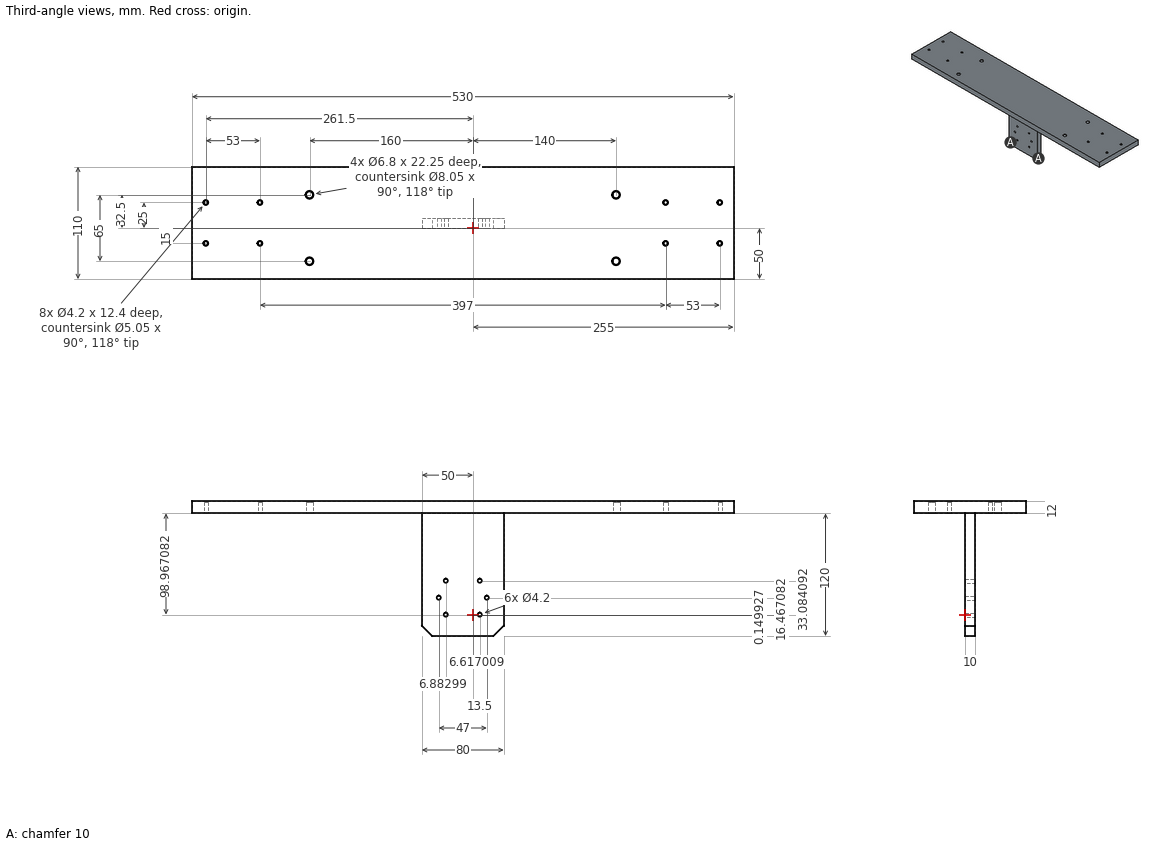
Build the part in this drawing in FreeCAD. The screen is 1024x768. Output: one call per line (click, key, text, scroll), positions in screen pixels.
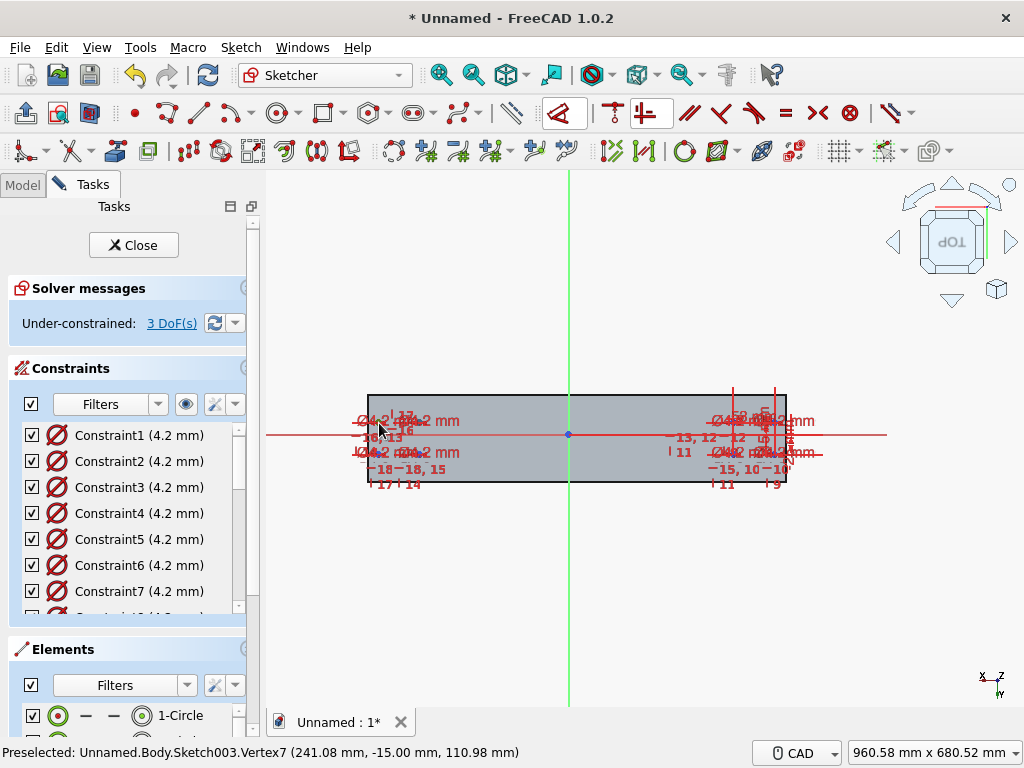
key(l)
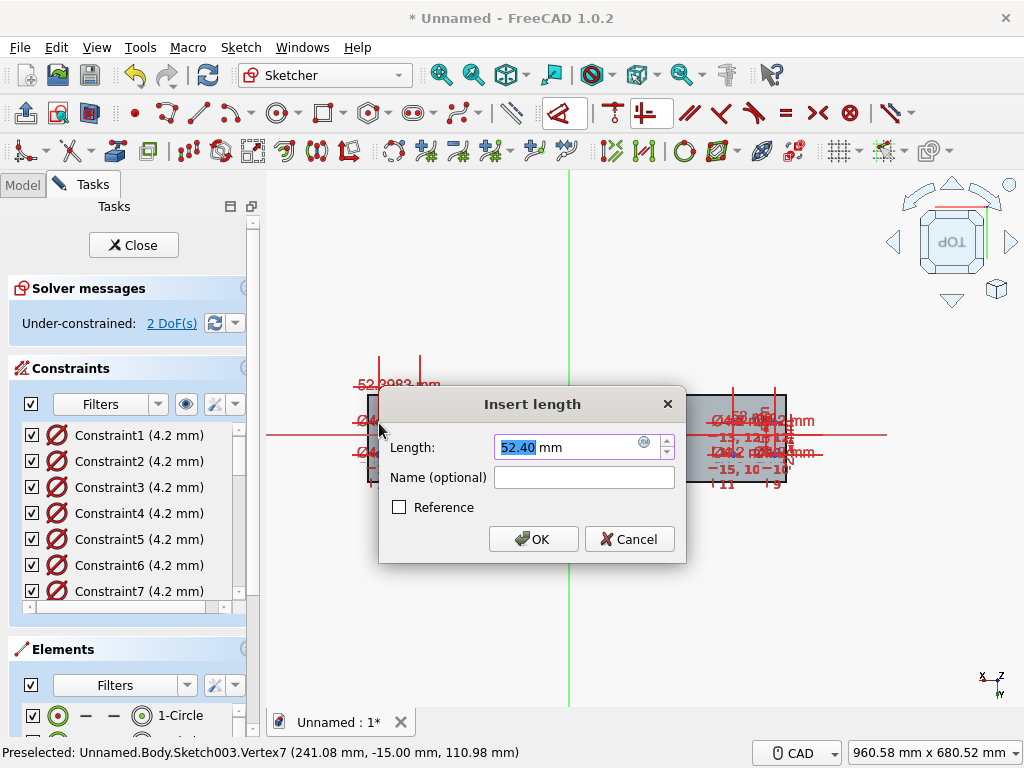
text(53)
key(Return)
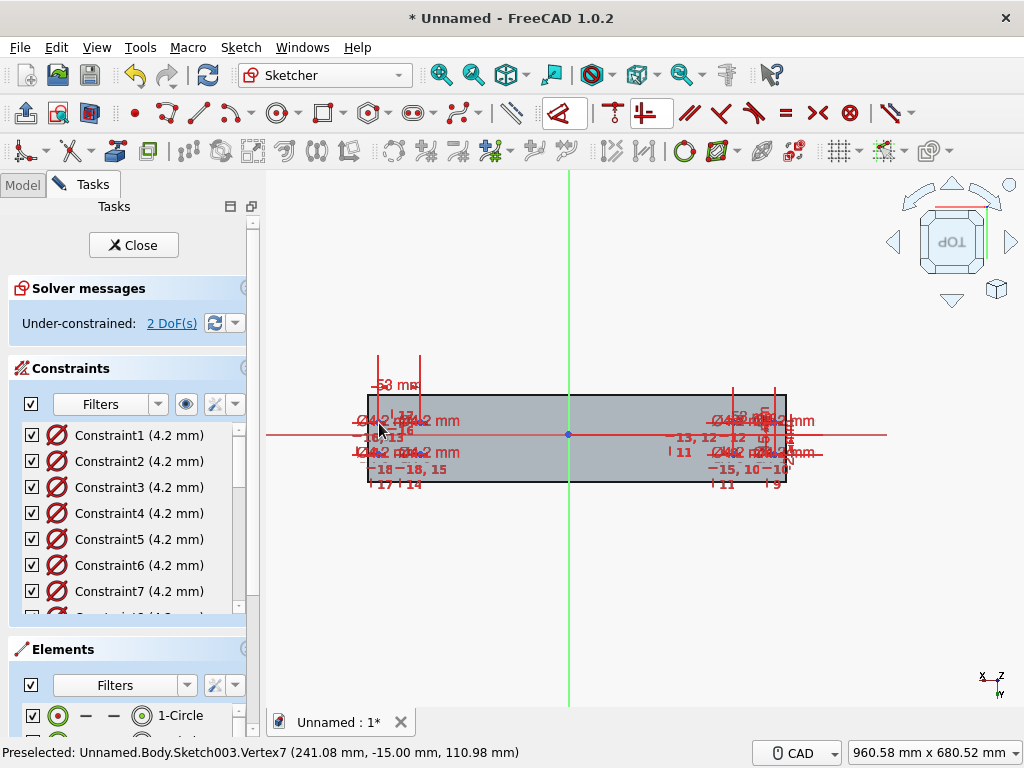
click(733, 423)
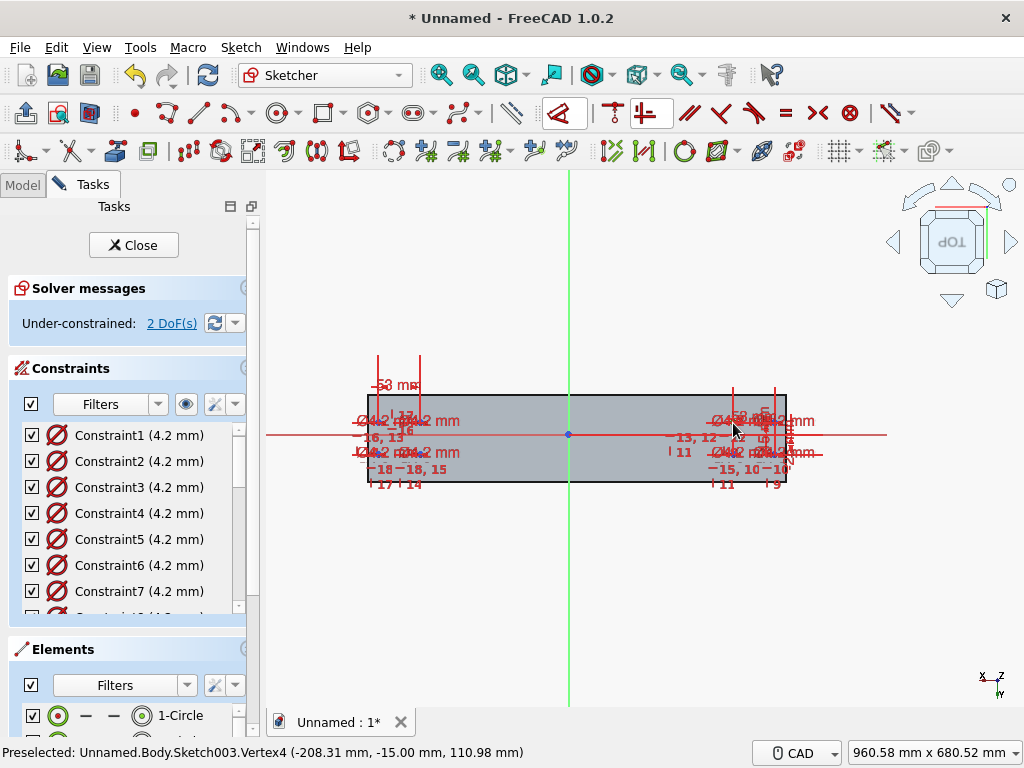
click(420, 423)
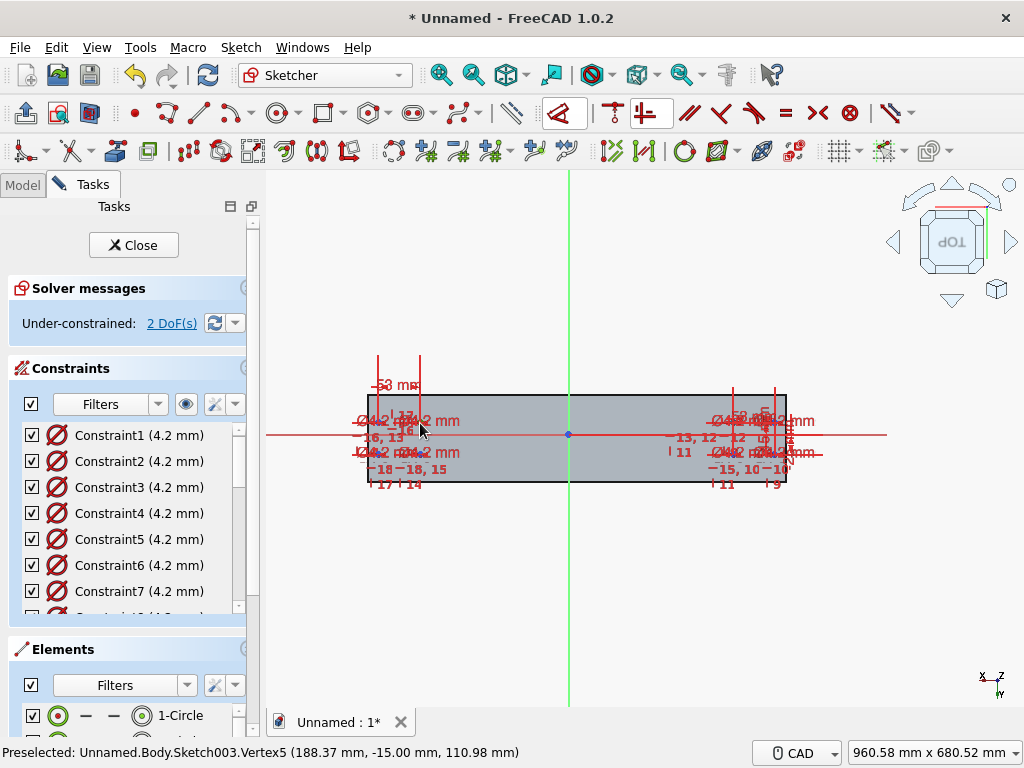
key(l)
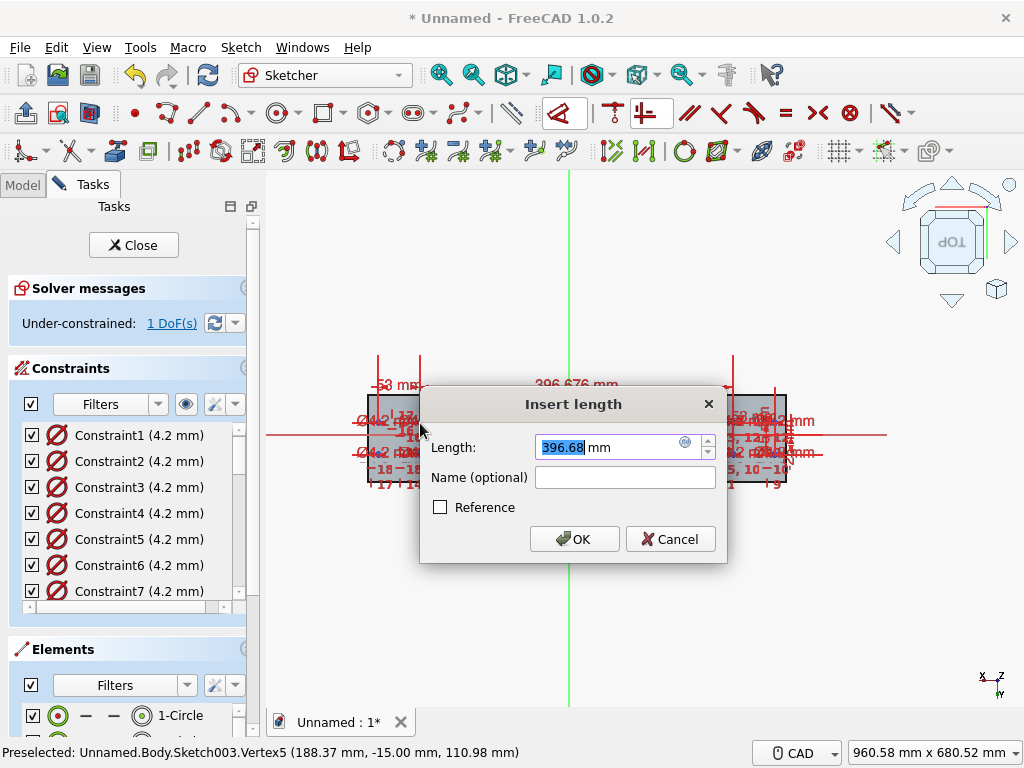
text(397)
key(Return)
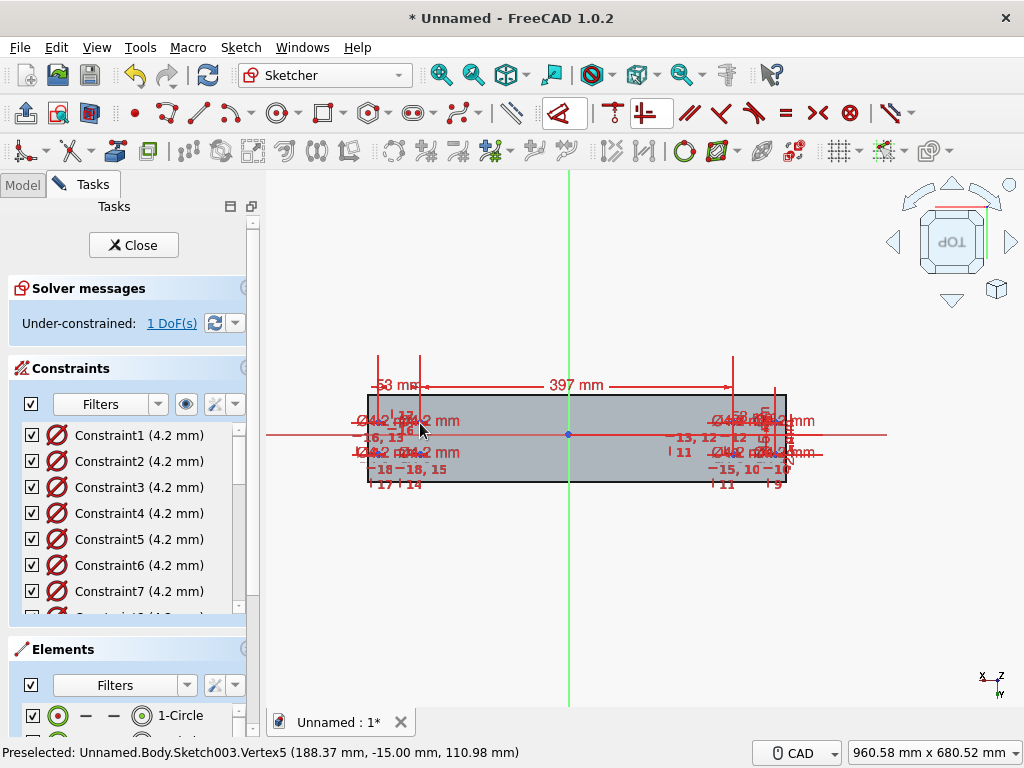
click(775, 455)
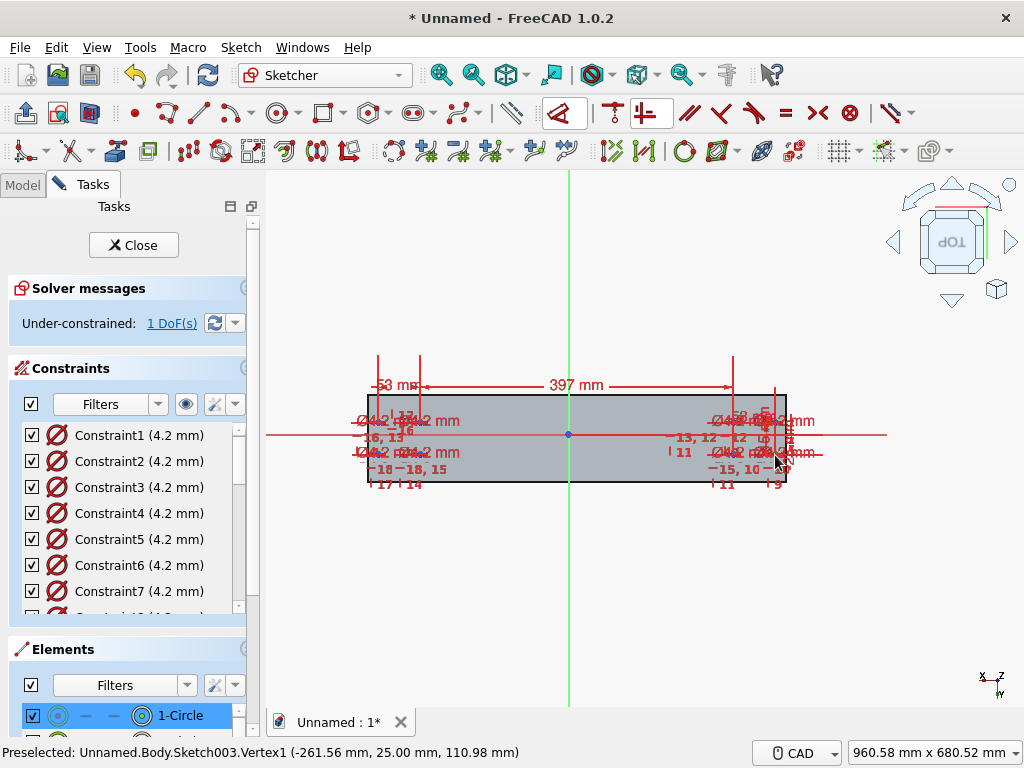
click(582, 114)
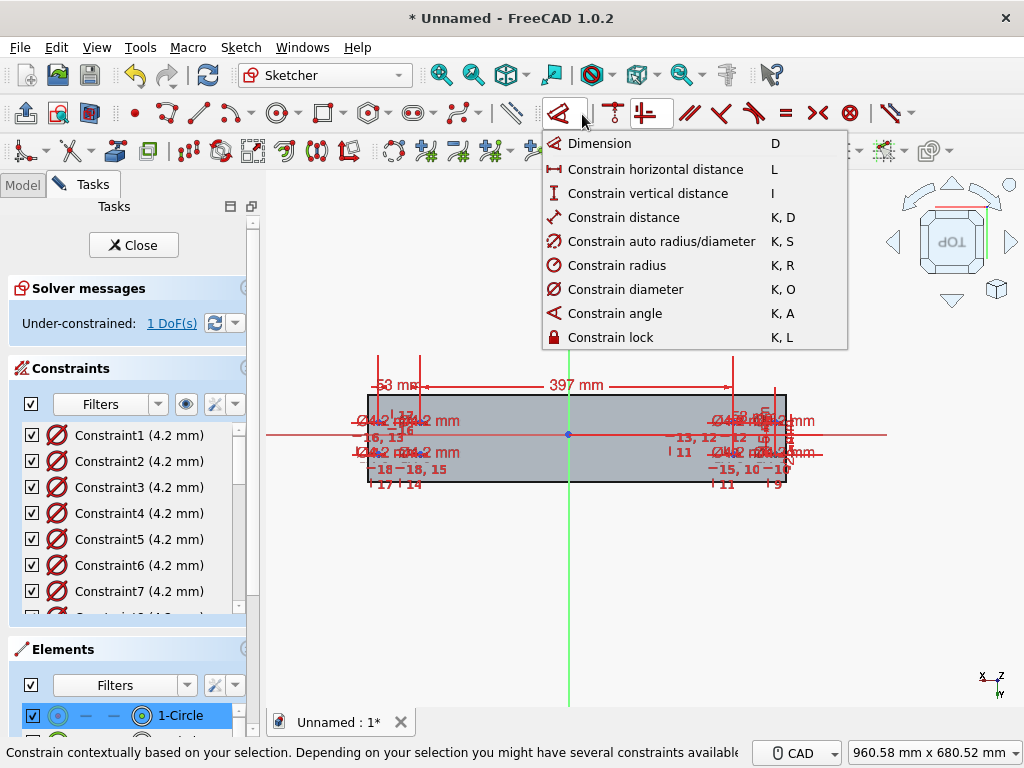
click(695, 169)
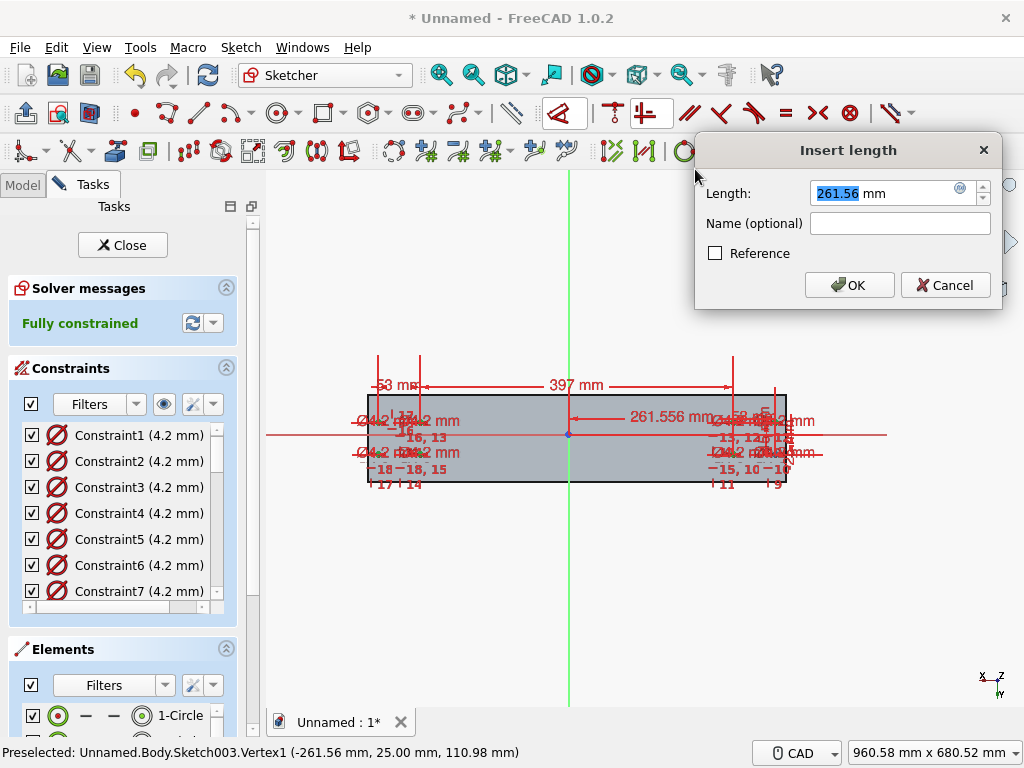
text(261.5)
key(Return)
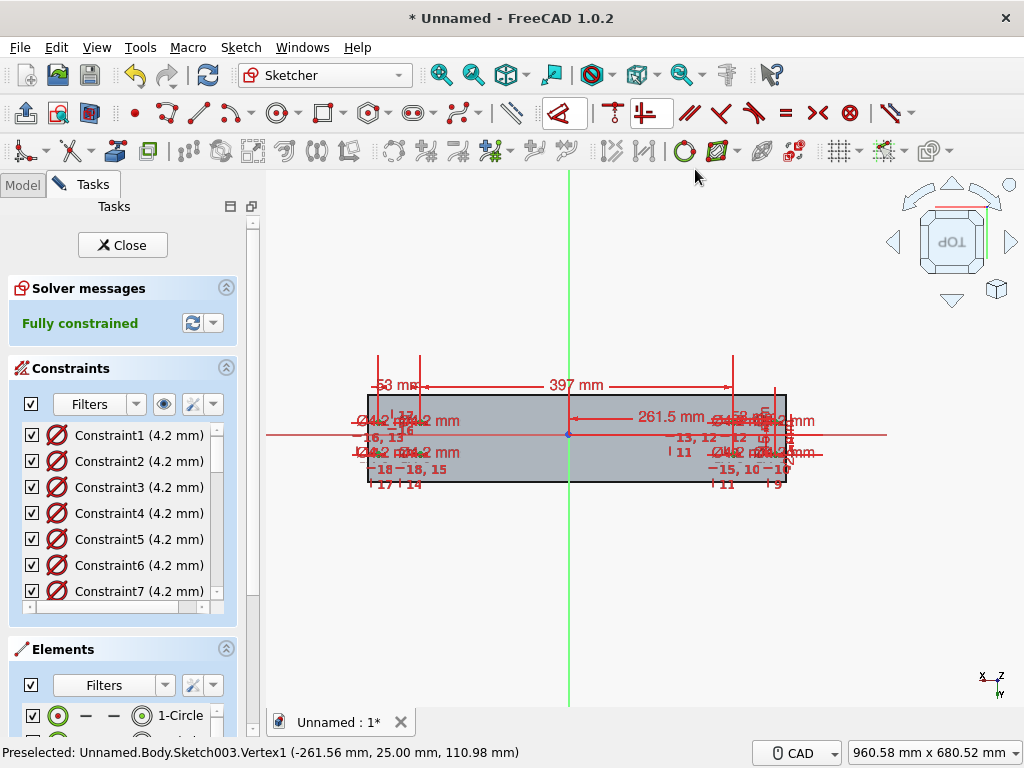
click(123, 245)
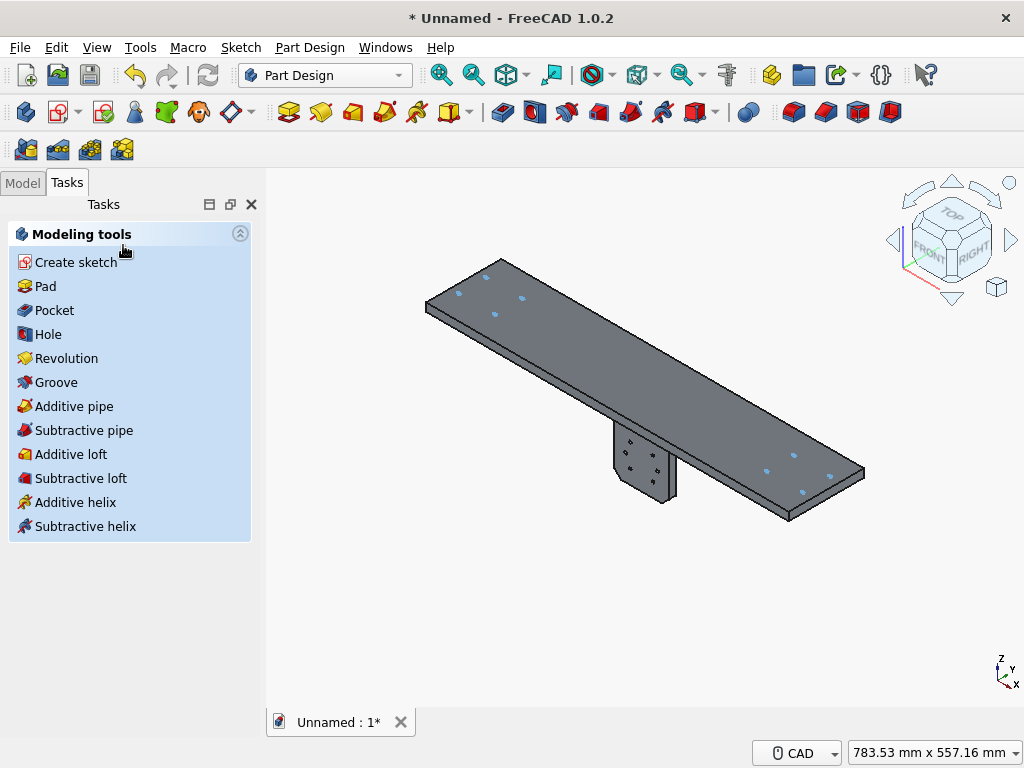
click(536, 112)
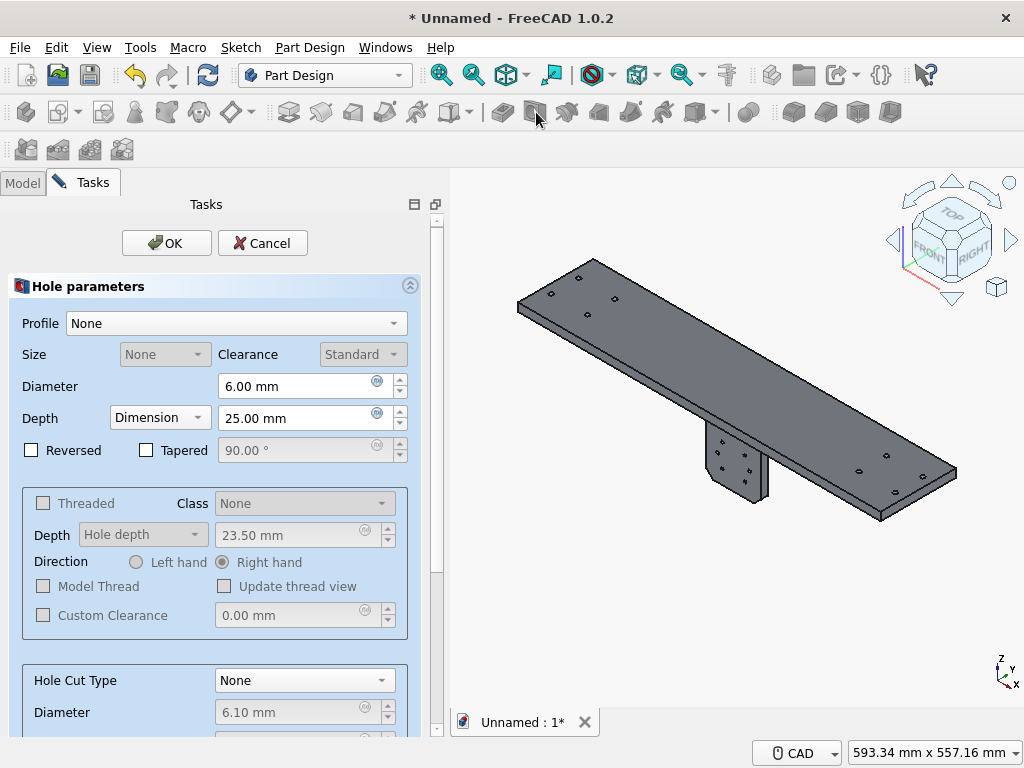
triple_click(305, 386)